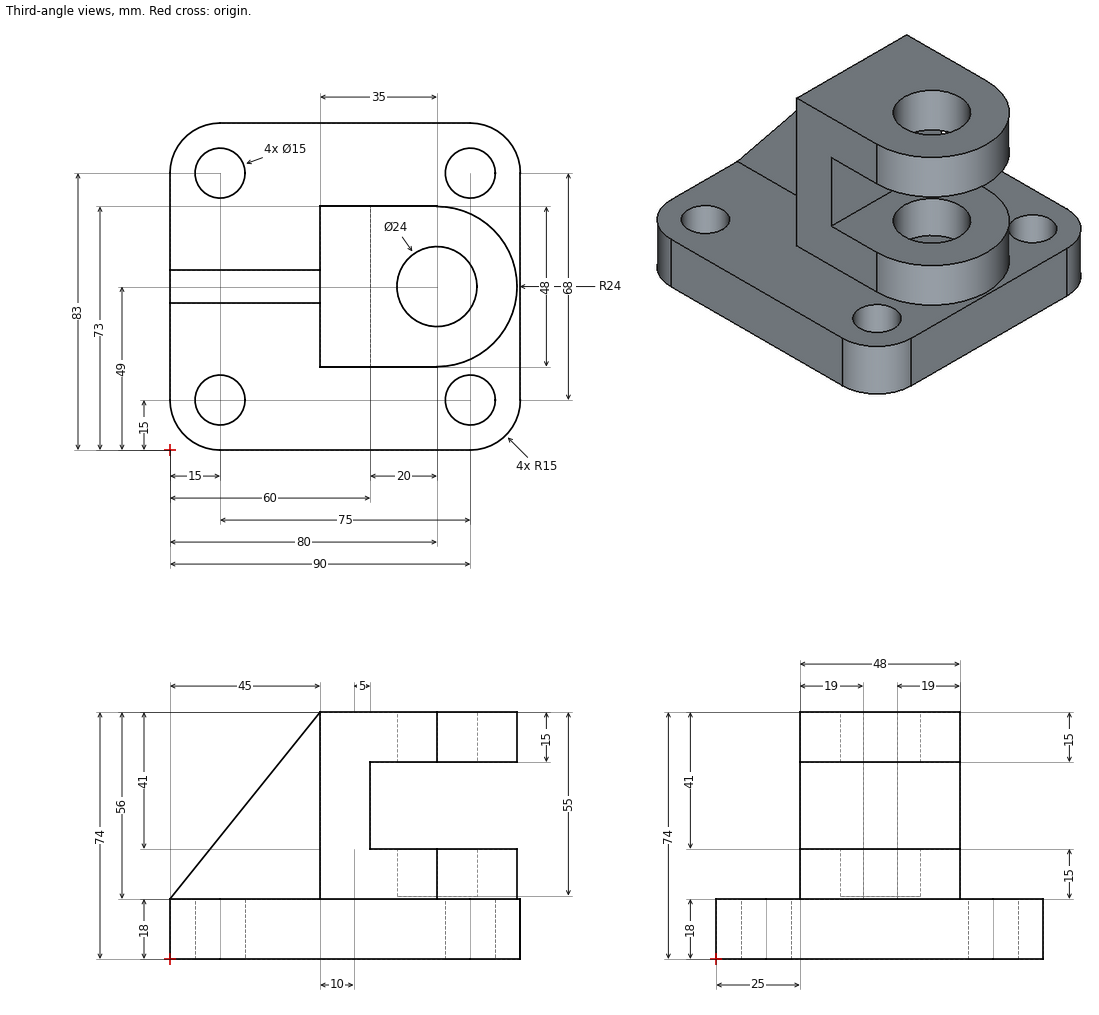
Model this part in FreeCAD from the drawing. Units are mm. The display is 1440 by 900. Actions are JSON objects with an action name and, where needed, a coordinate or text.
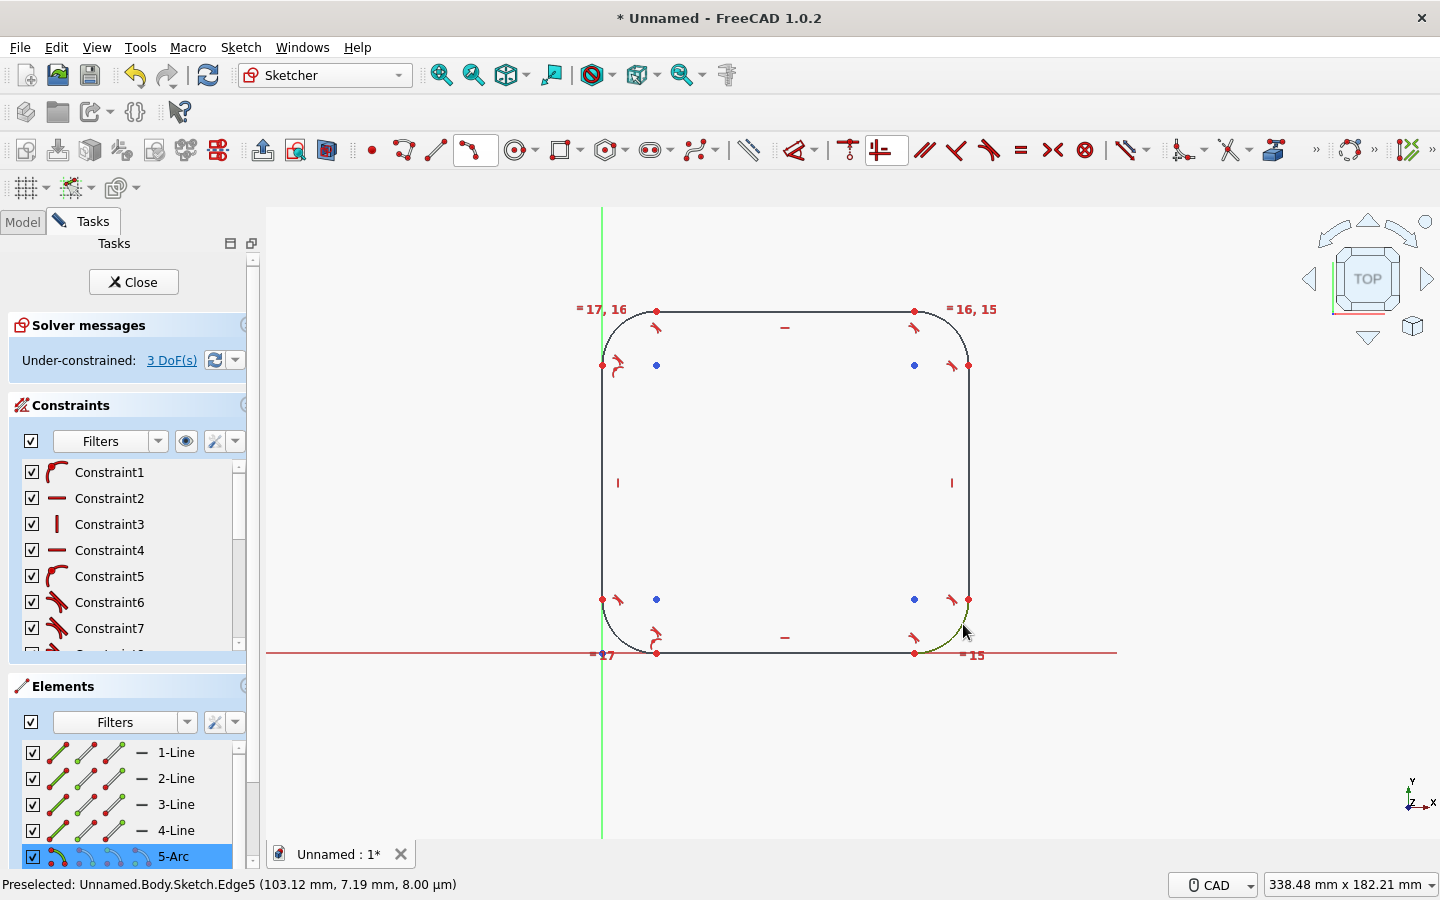
{"action": "key", "text": "k r"}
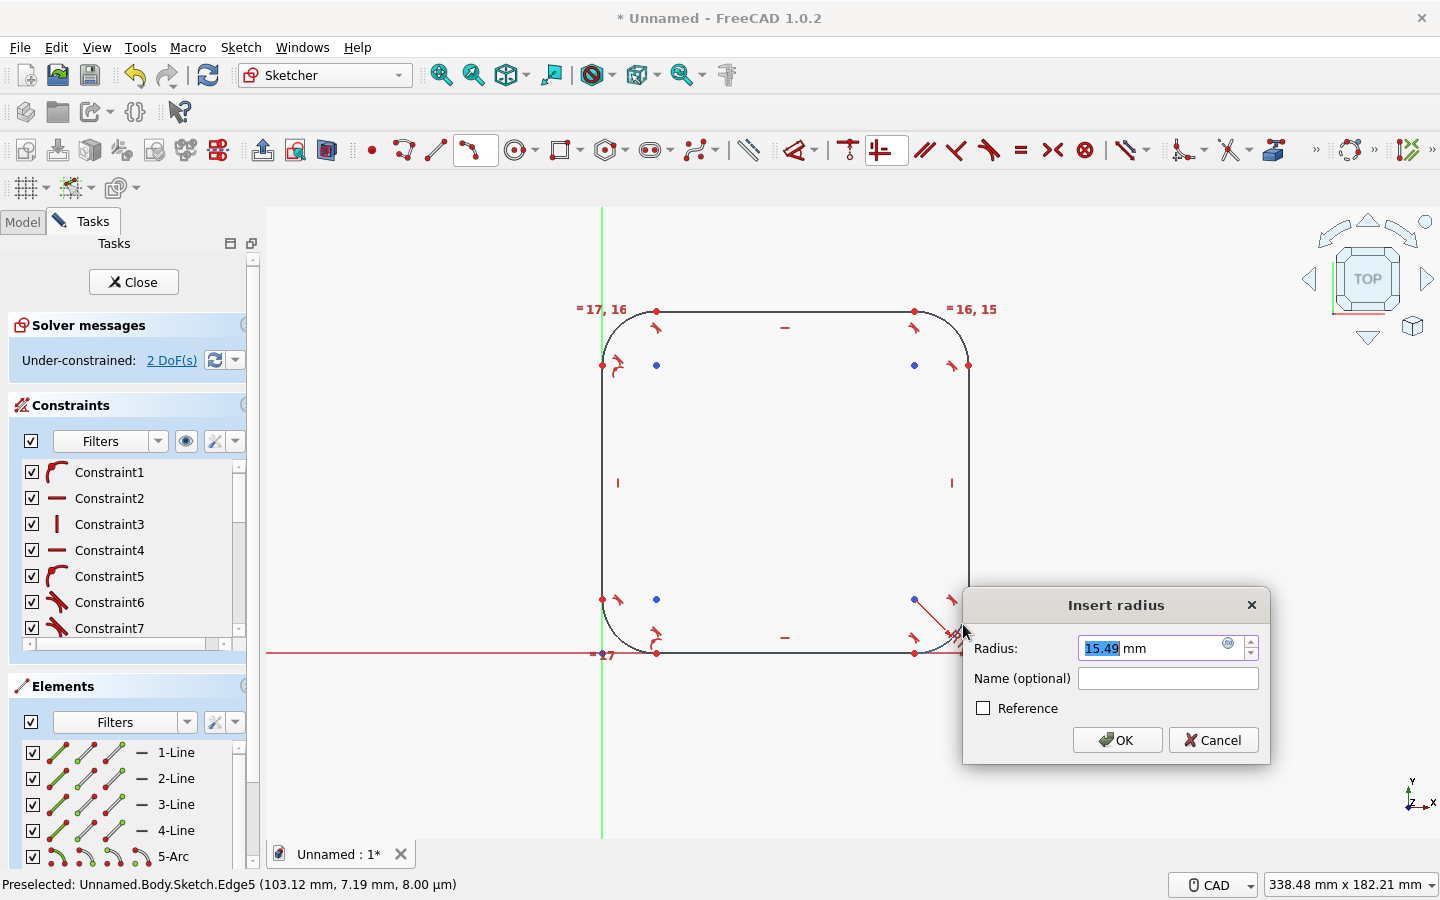
{"action": "type", "text": "15"}
{"action": "key", "text": "Return"}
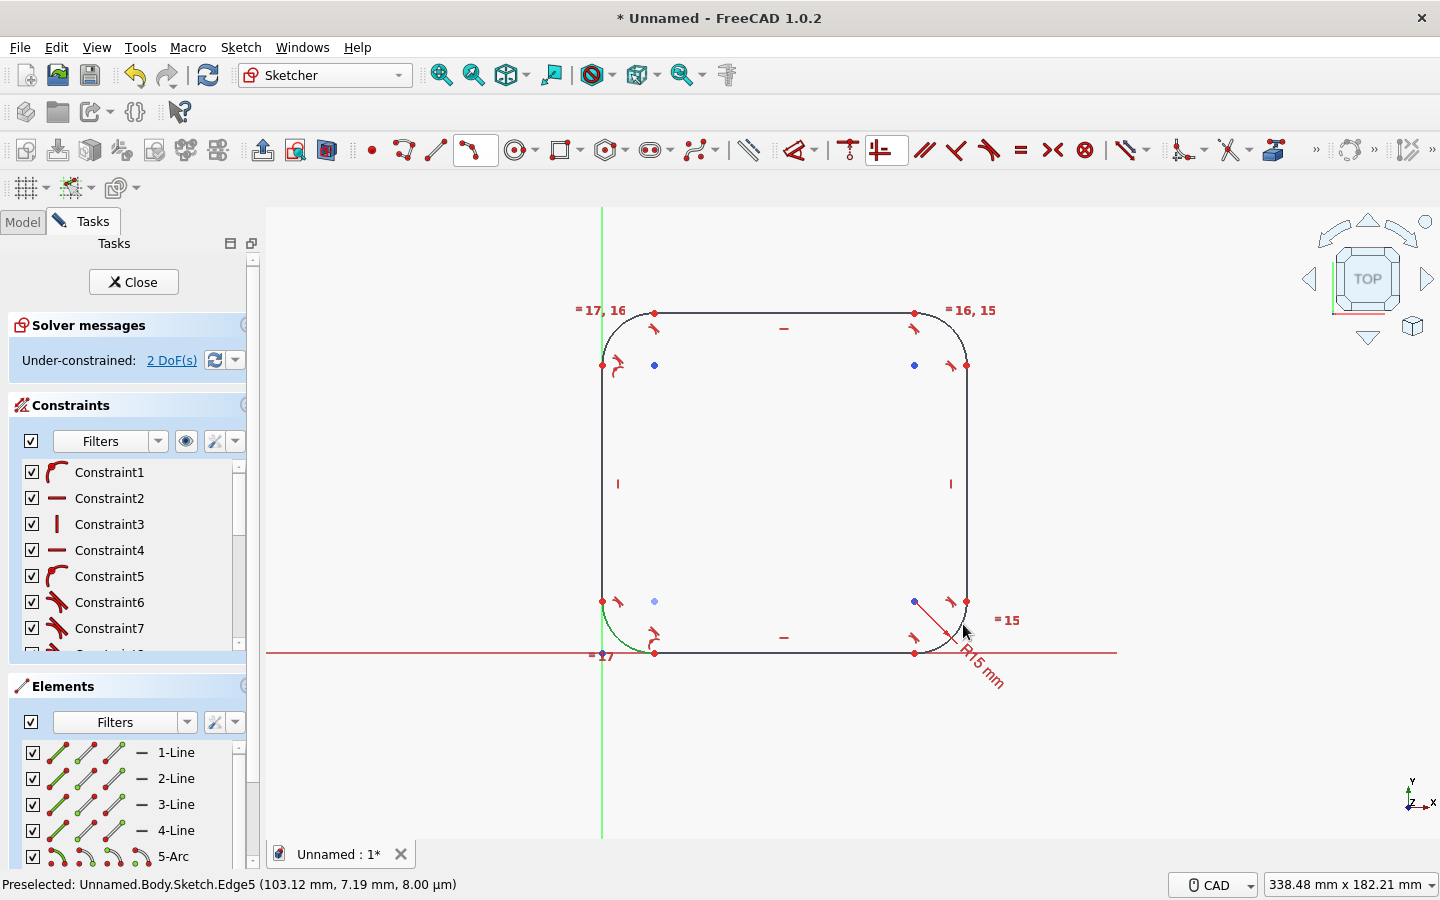
{"action": "left_click", "coordinate": [733, 653]}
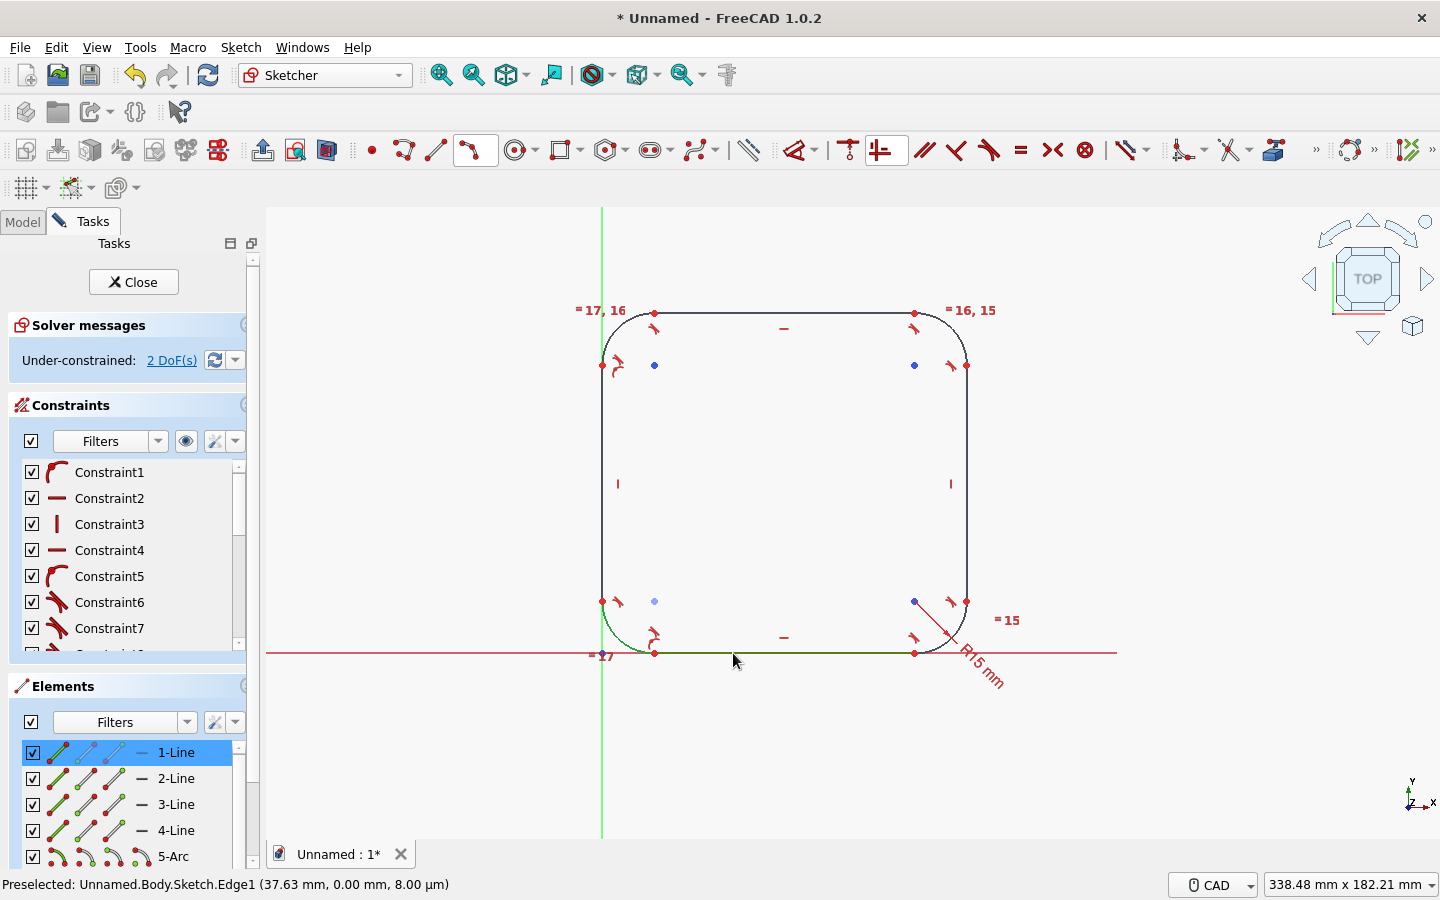
{"action": "left_click", "coordinate": [816, 150]}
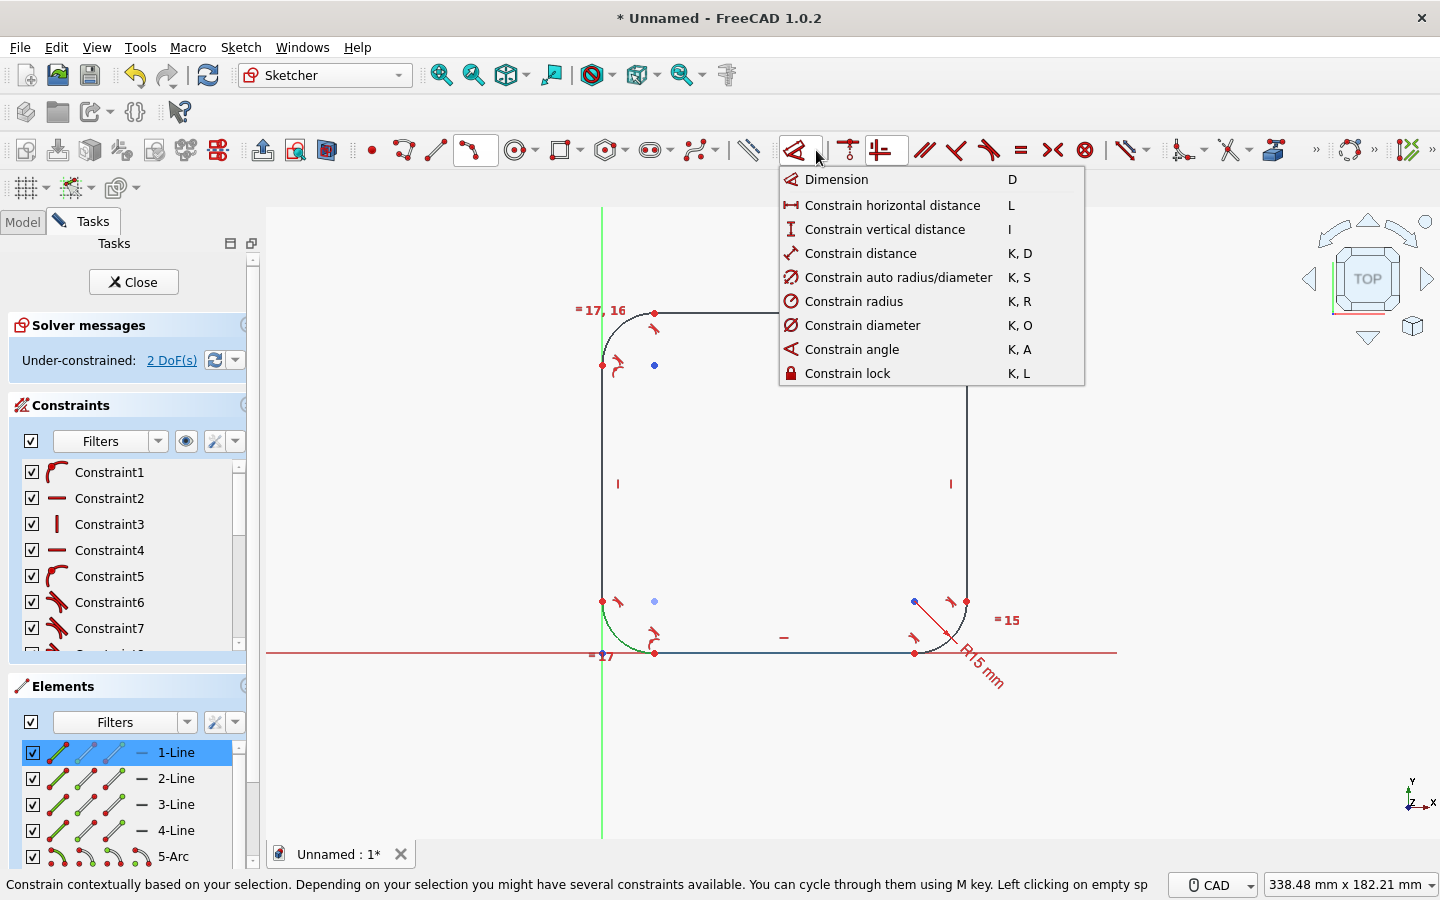
{"action": "left_click", "coordinate": [932, 205]}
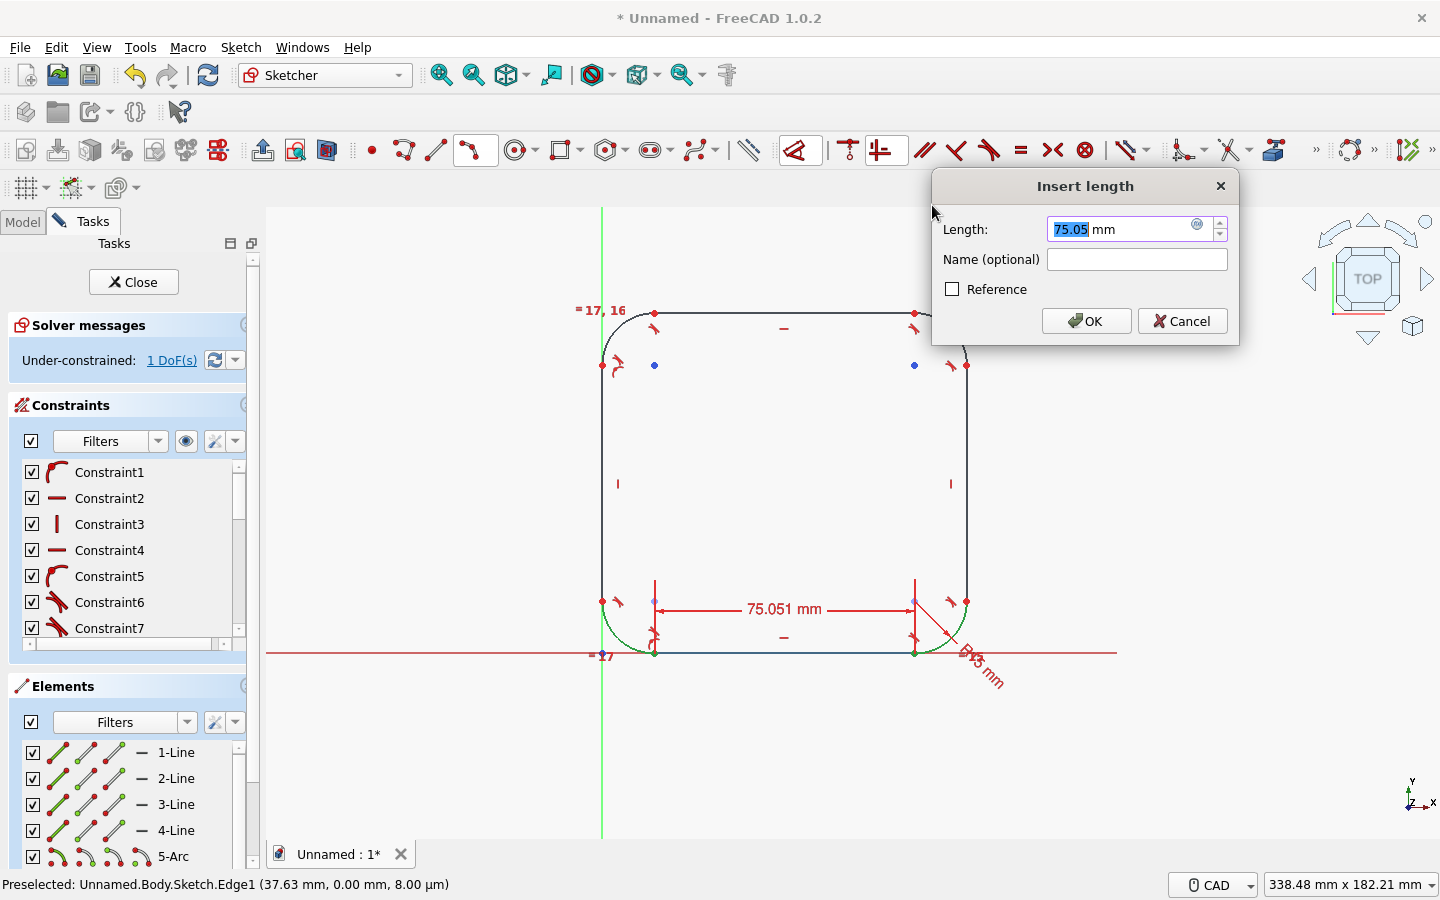
{"action": "type", "text": "75"}
{"action": "key", "text": "Return"}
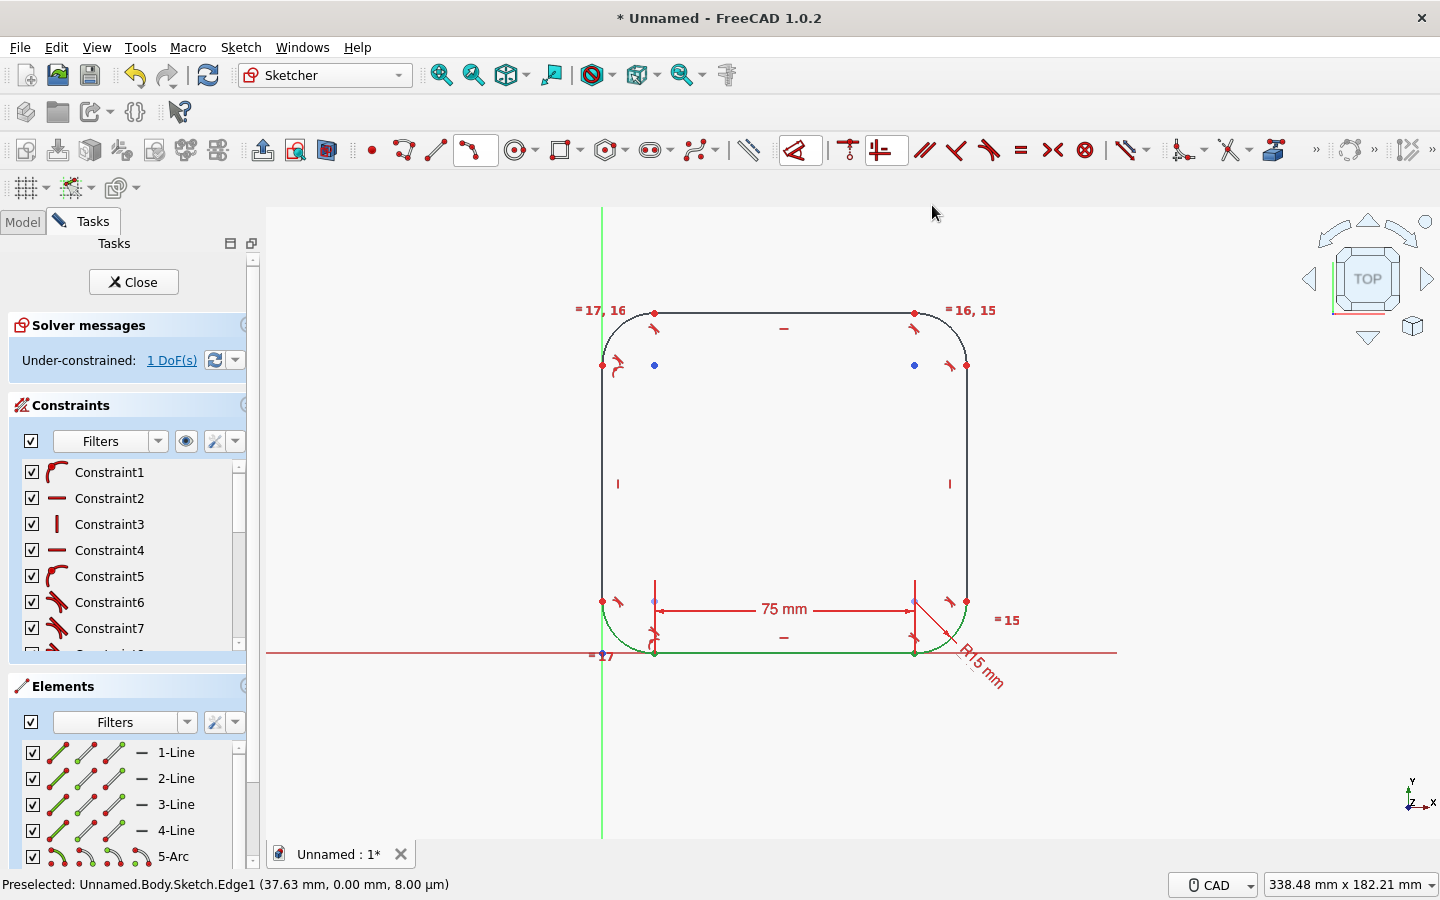
{"action": "left_click", "coordinate": [967, 531]}